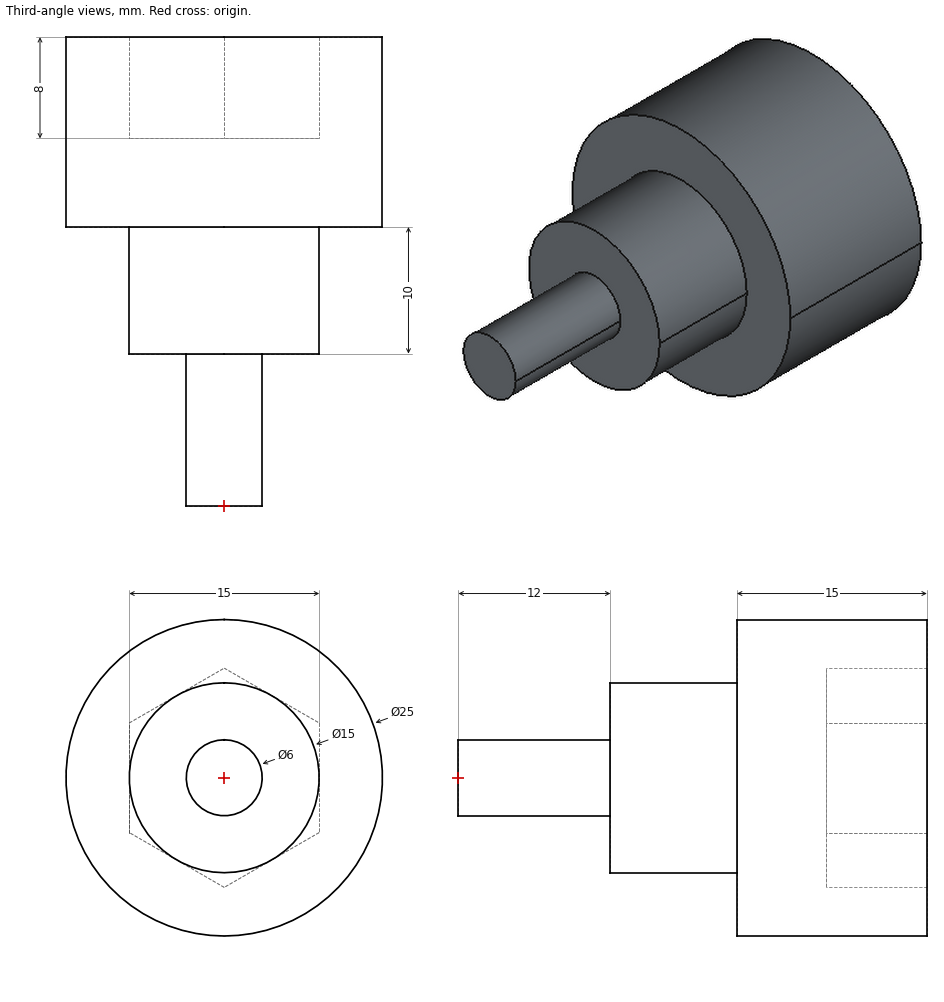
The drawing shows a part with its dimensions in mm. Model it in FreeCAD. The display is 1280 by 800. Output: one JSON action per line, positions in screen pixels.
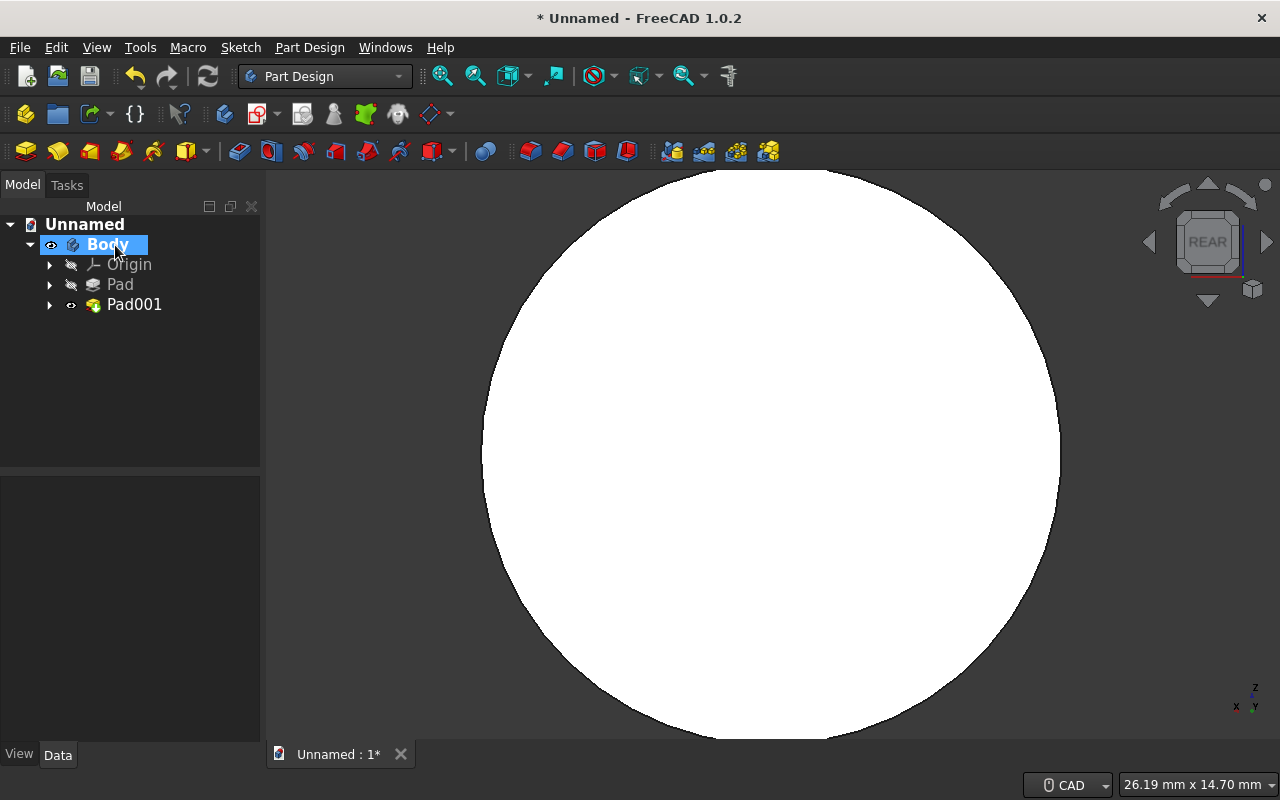
{"action": "key", "text": "v f"}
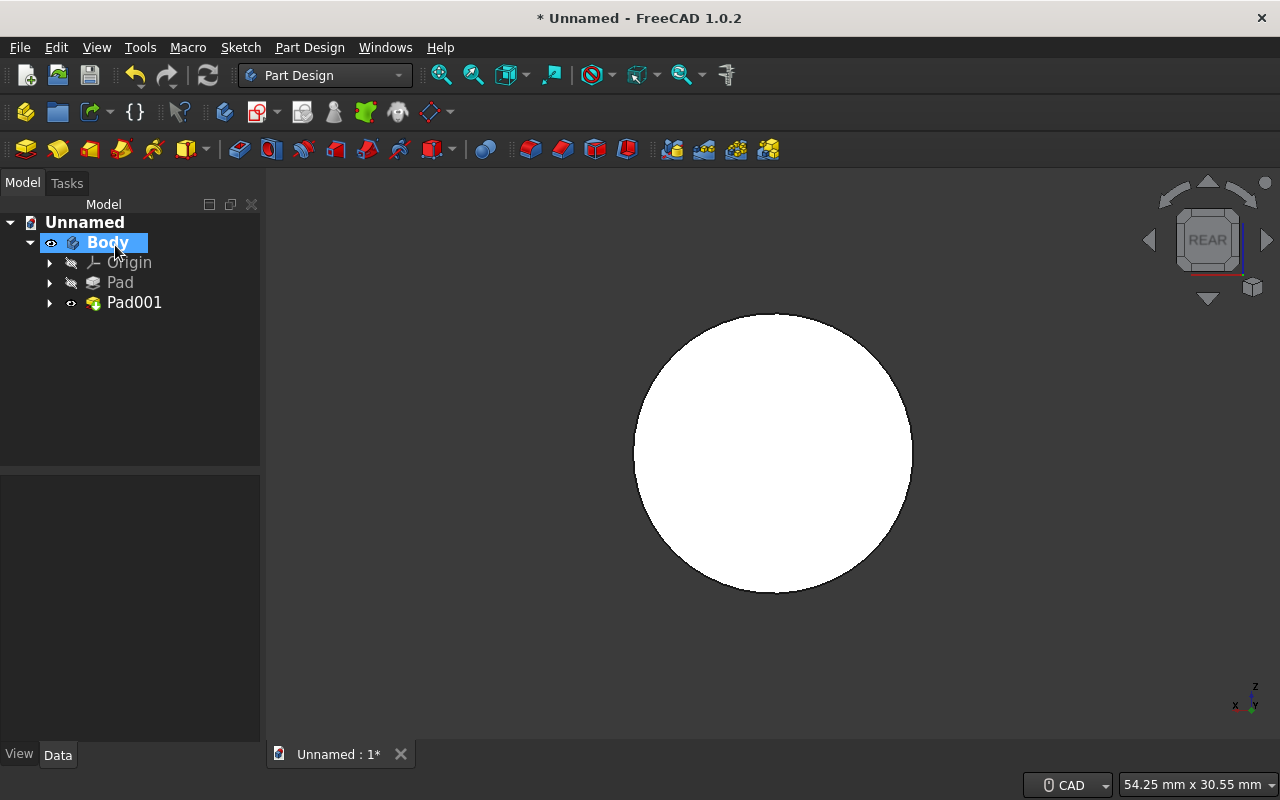
{"action": "left_click", "coordinate": [773, 452]}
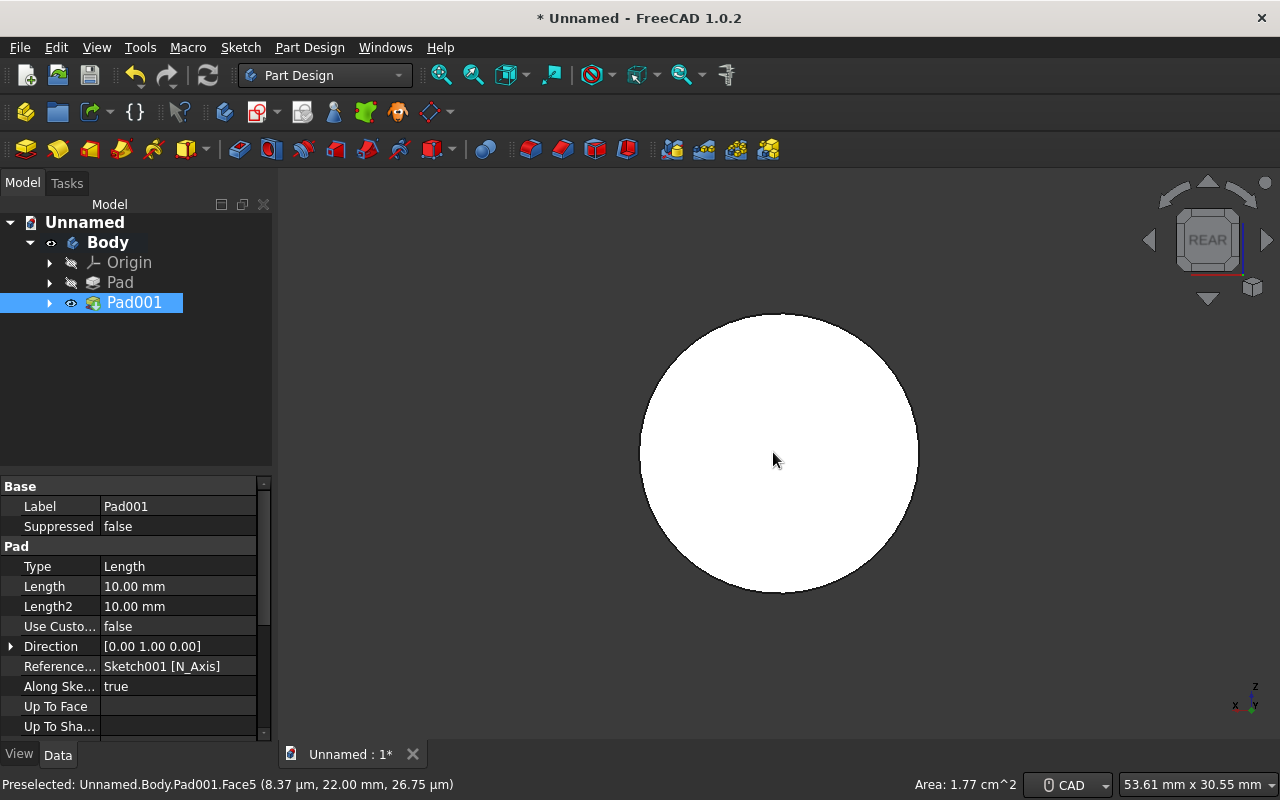
{"action": "left_click", "coordinate": [258, 112]}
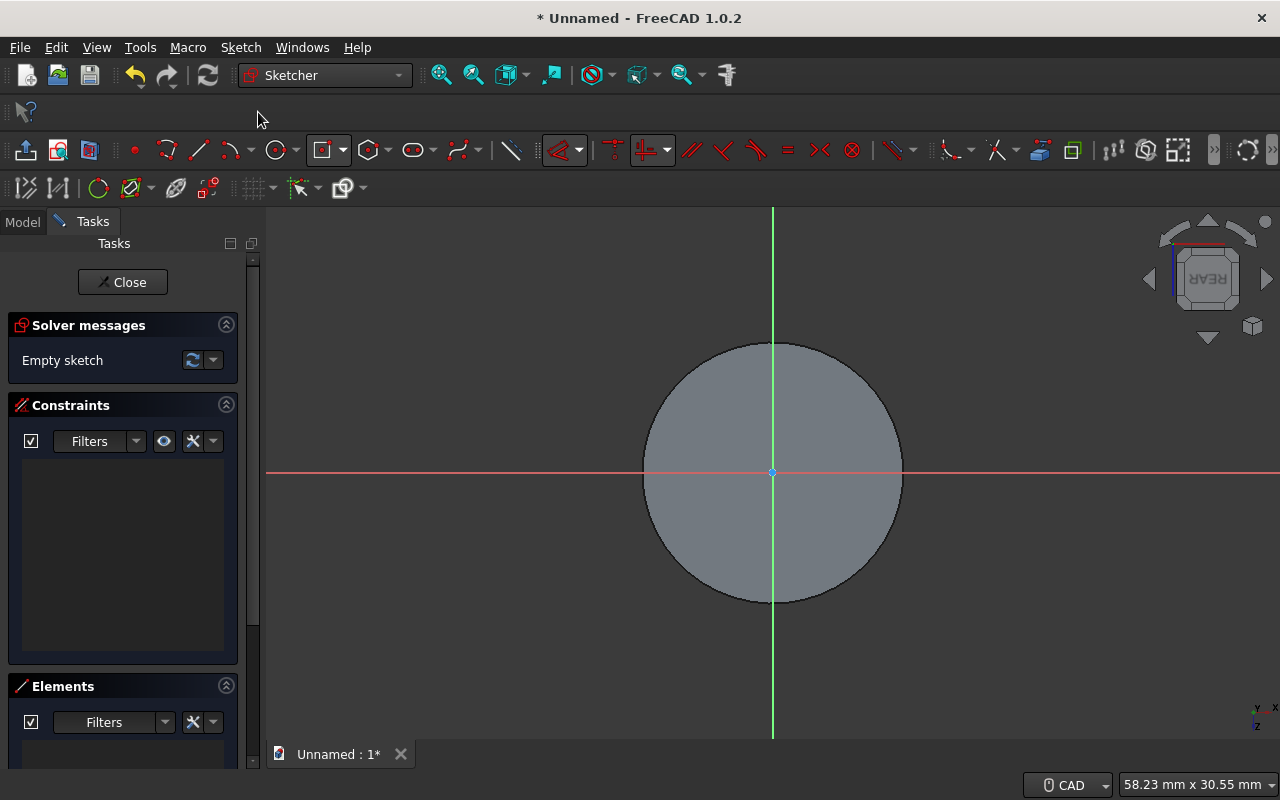
{"action": "scroll", "coordinate": [396, 473], "scroll_direction": "down", "scroll_amount": 1}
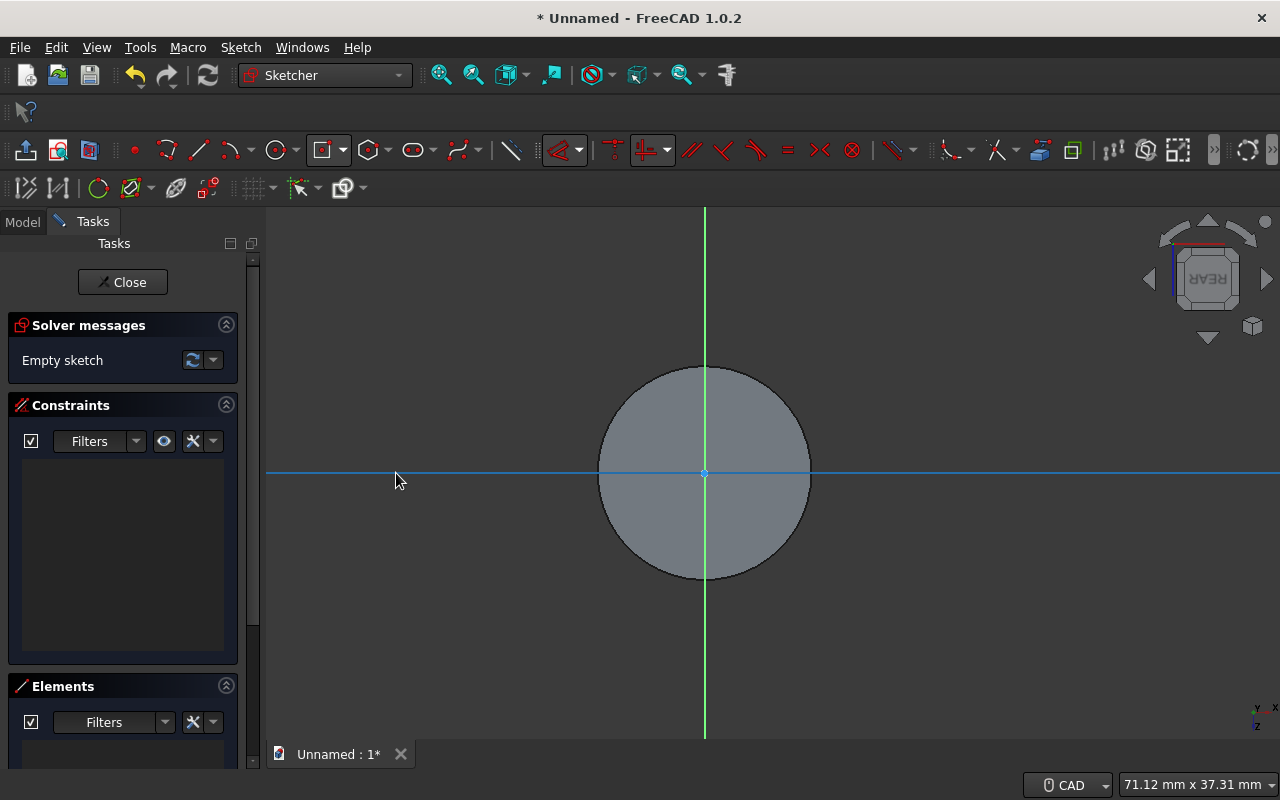
{"action": "key", "text": "g c"}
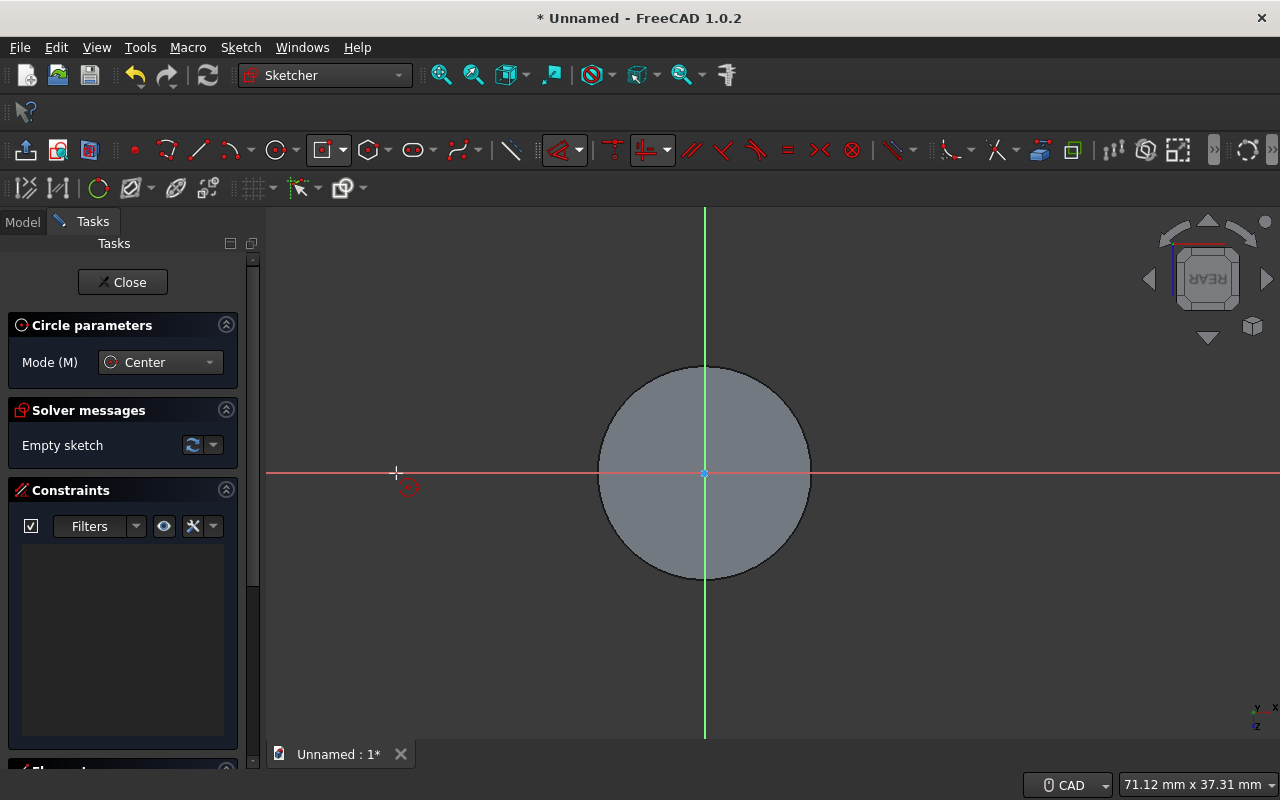
{"action": "left_click", "coordinate": [705, 473]}
{"action": "left_click", "coordinate": [831, 347]}
{"action": "key", "text": "Escape"}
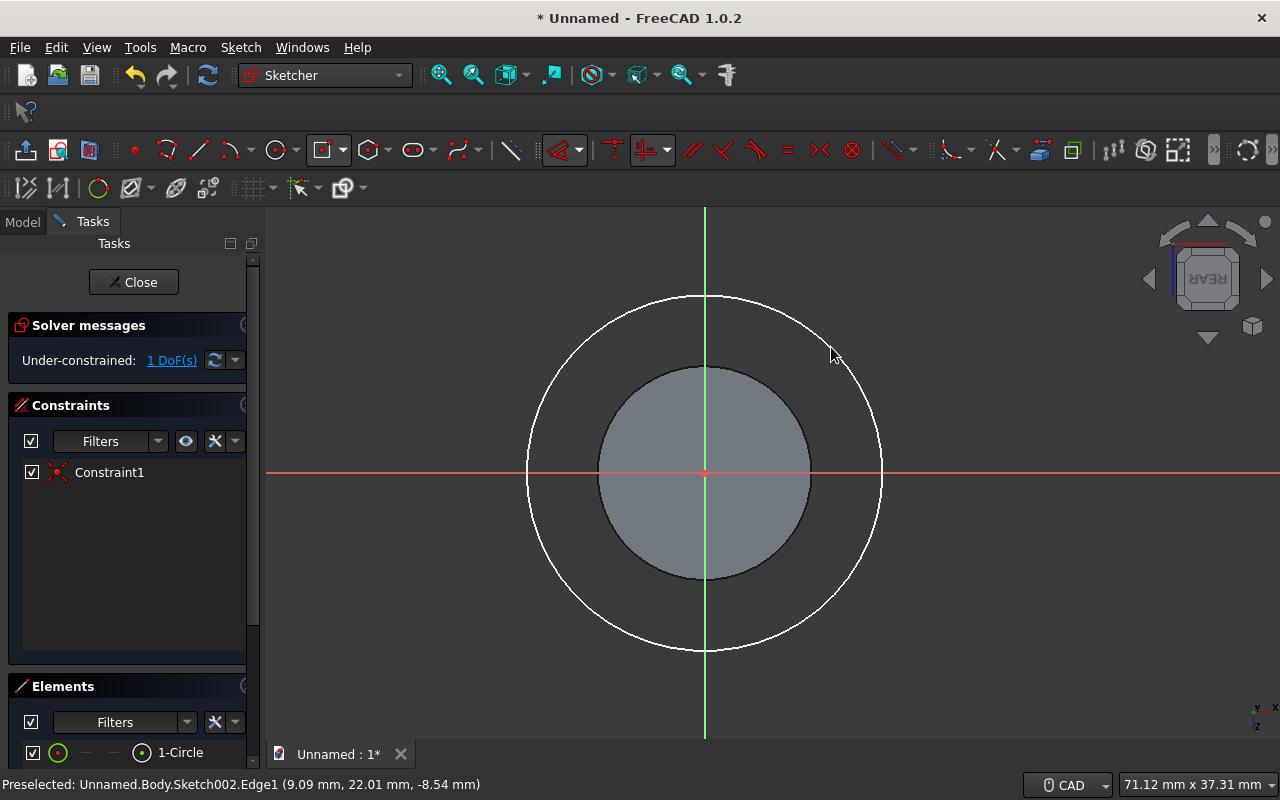
{"action": "left_click", "coordinate": [830, 347]}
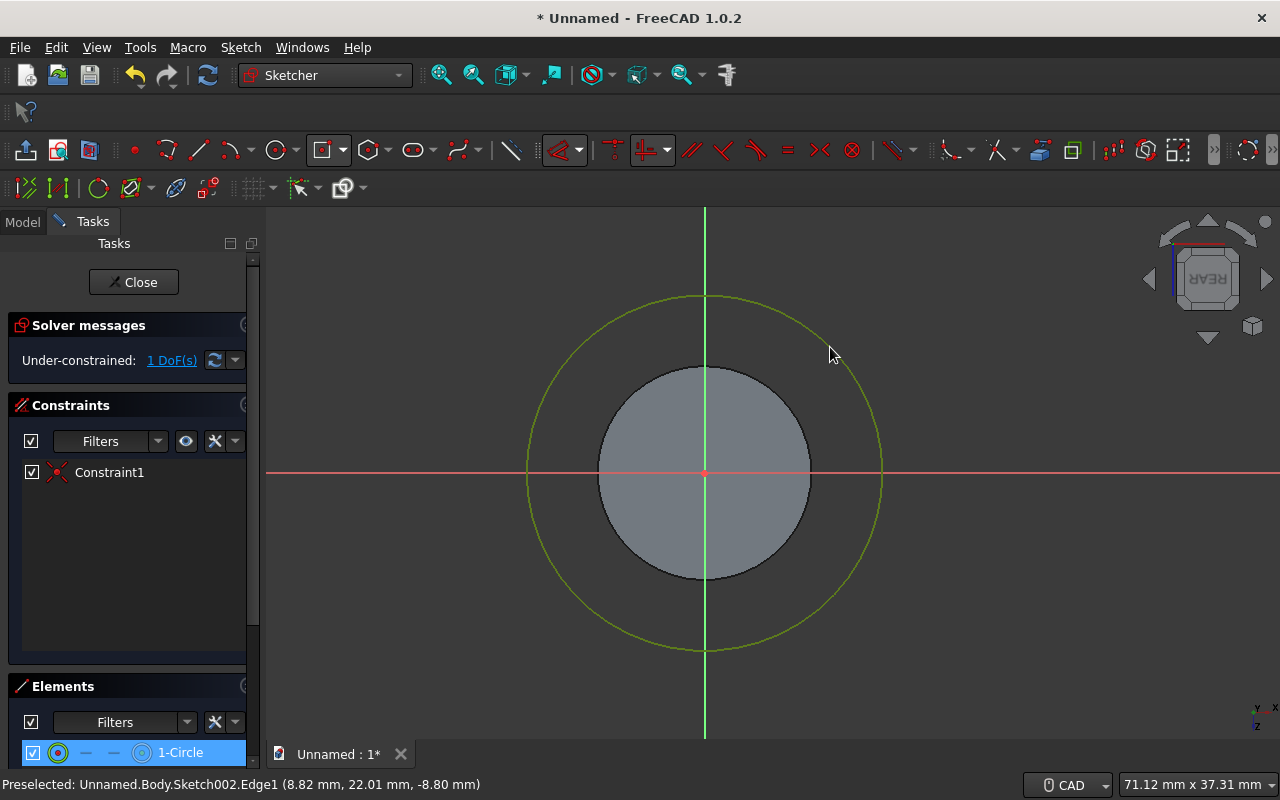
{"action": "key", "text": "k o"}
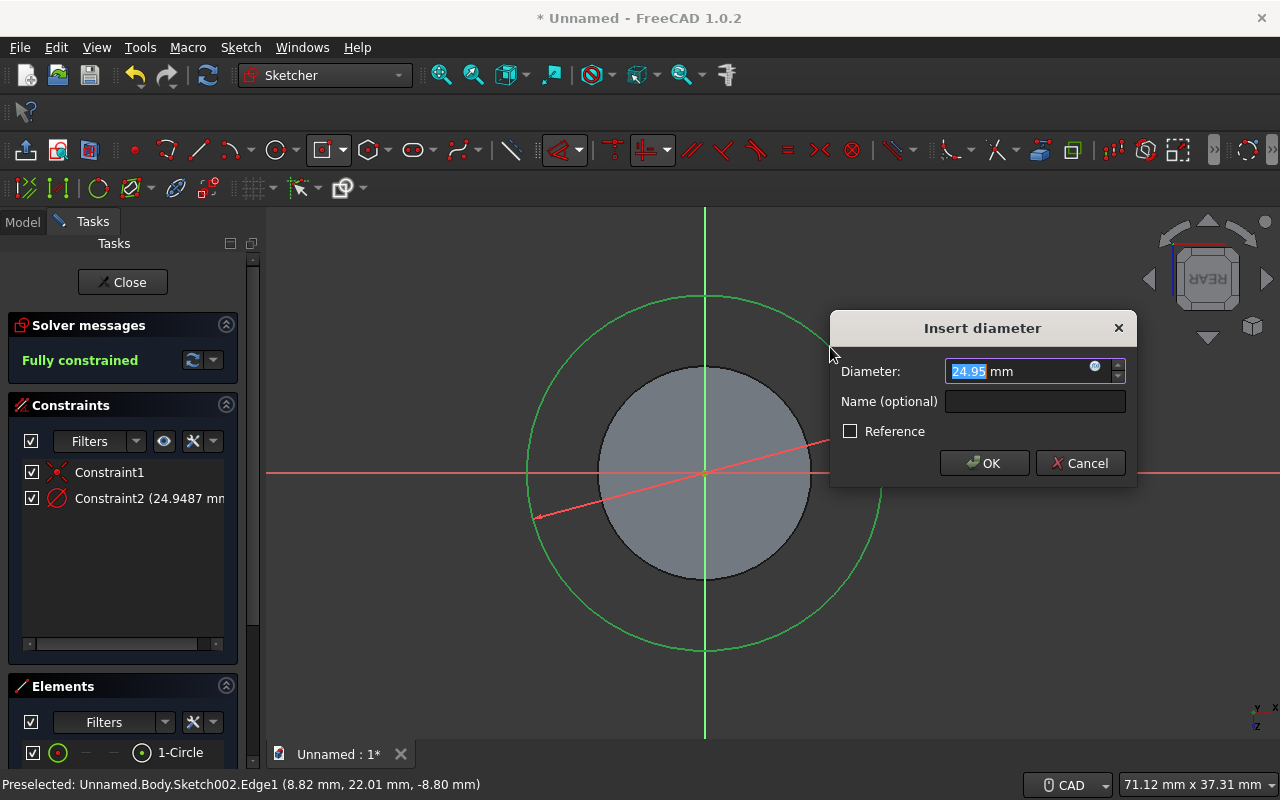
{"action": "type", "text": "25"}
{"action": "key", "text": "Return"}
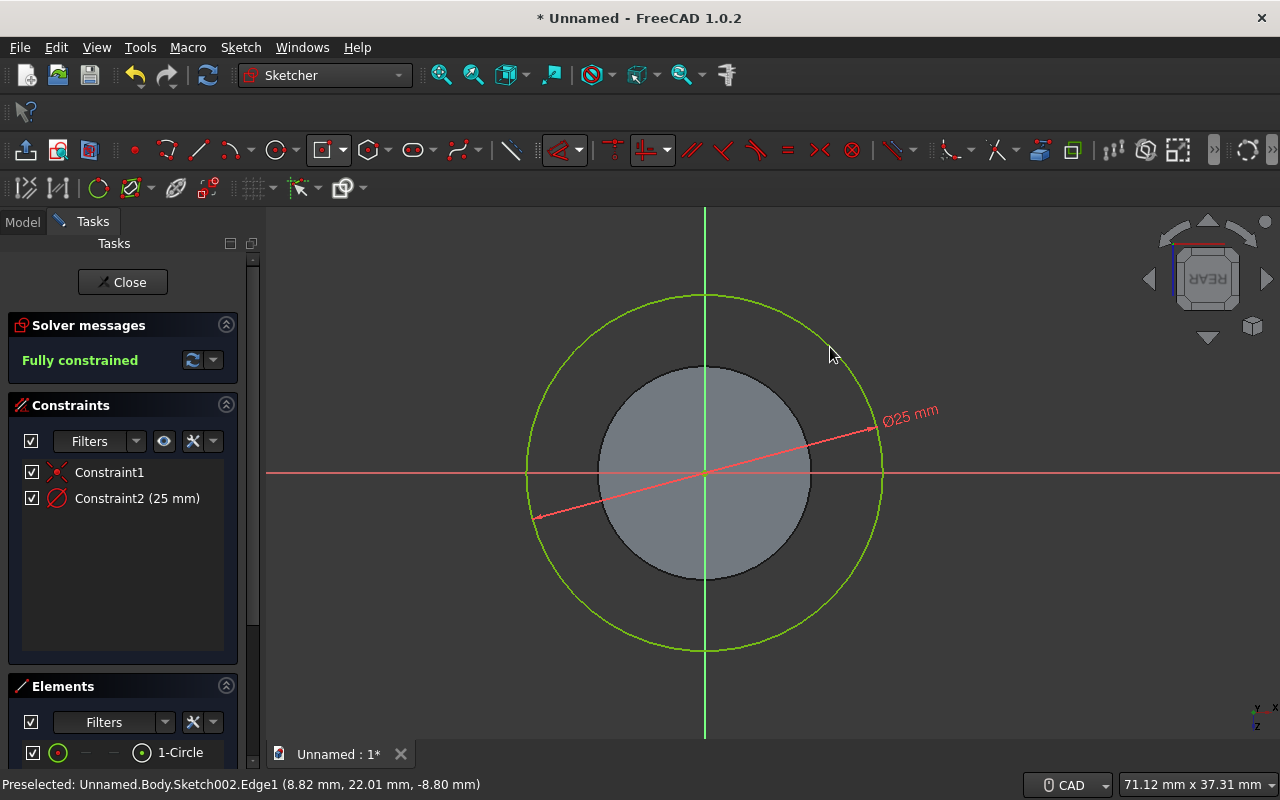
{"action": "left_click", "coordinate": [123, 282]}